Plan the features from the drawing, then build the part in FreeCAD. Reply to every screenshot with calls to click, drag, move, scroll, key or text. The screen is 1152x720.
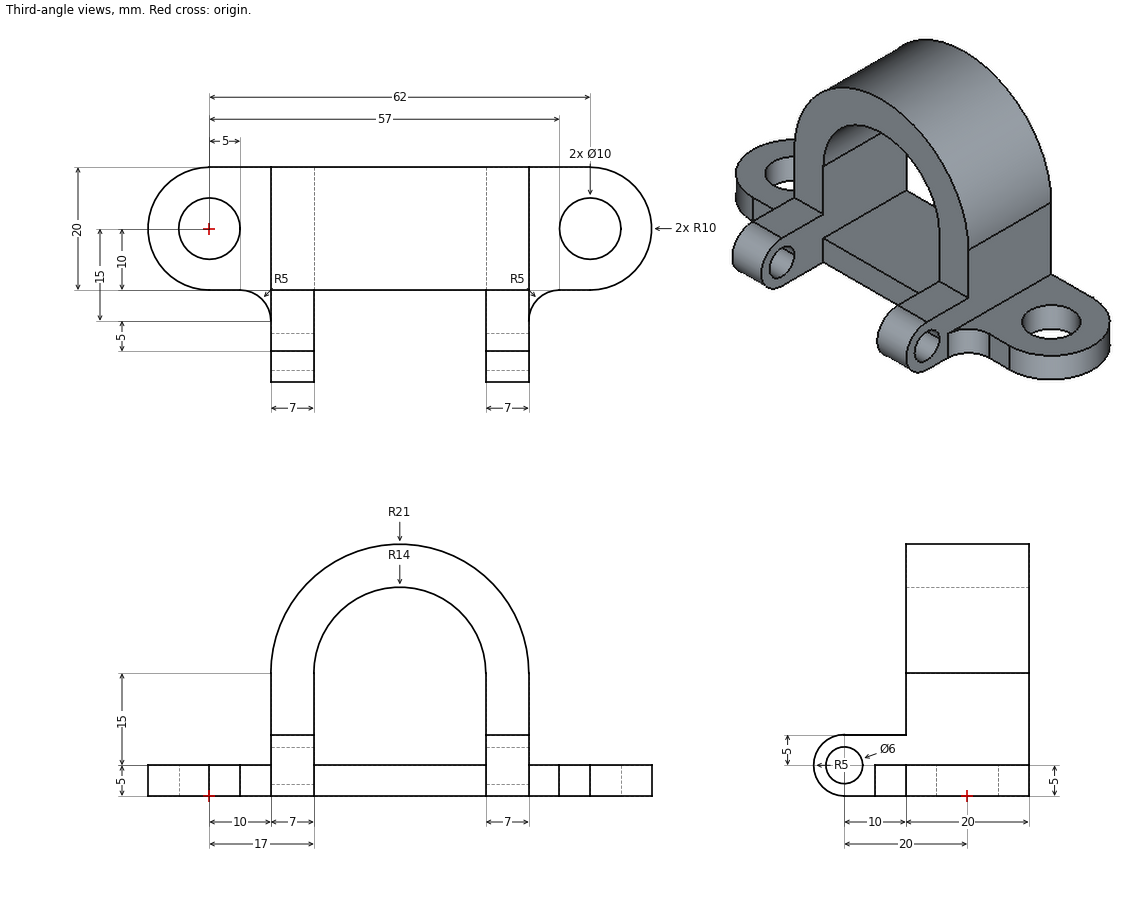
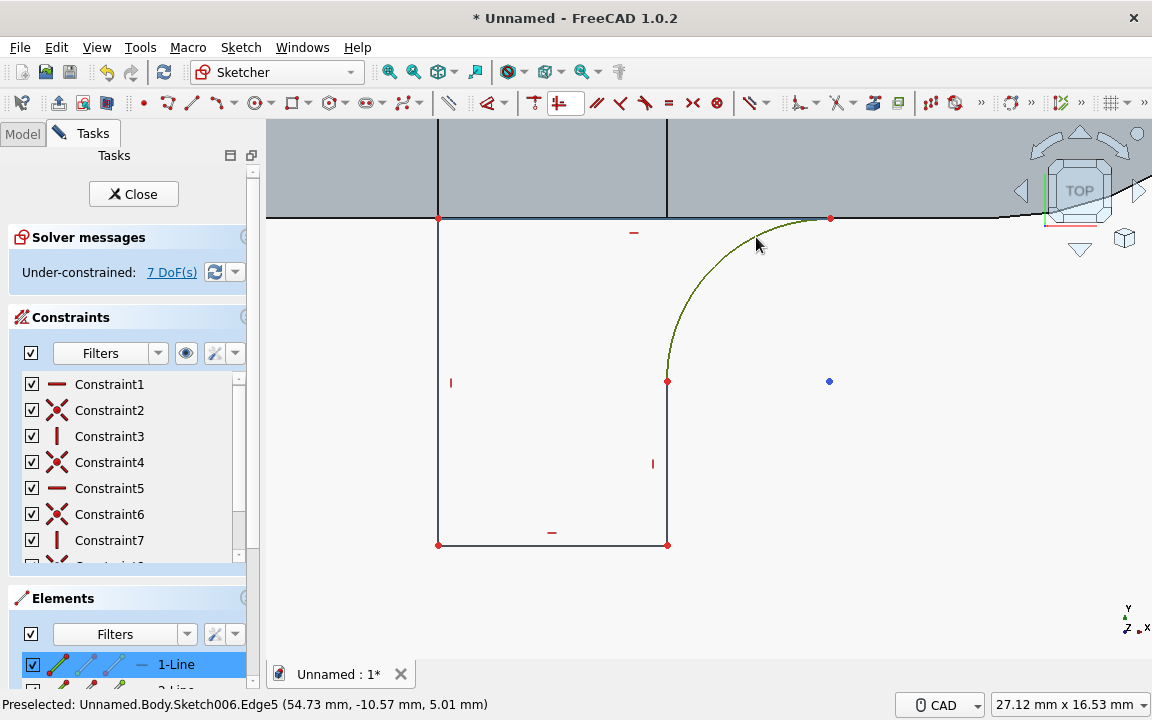
click(646, 104)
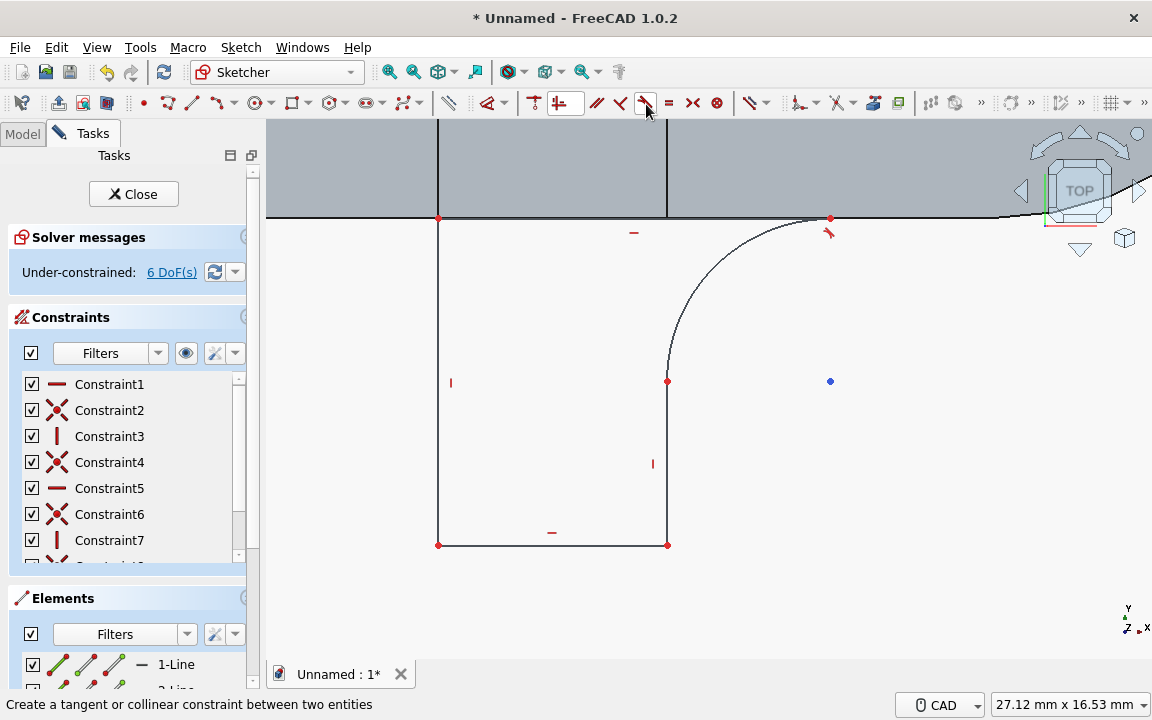
click(667, 497)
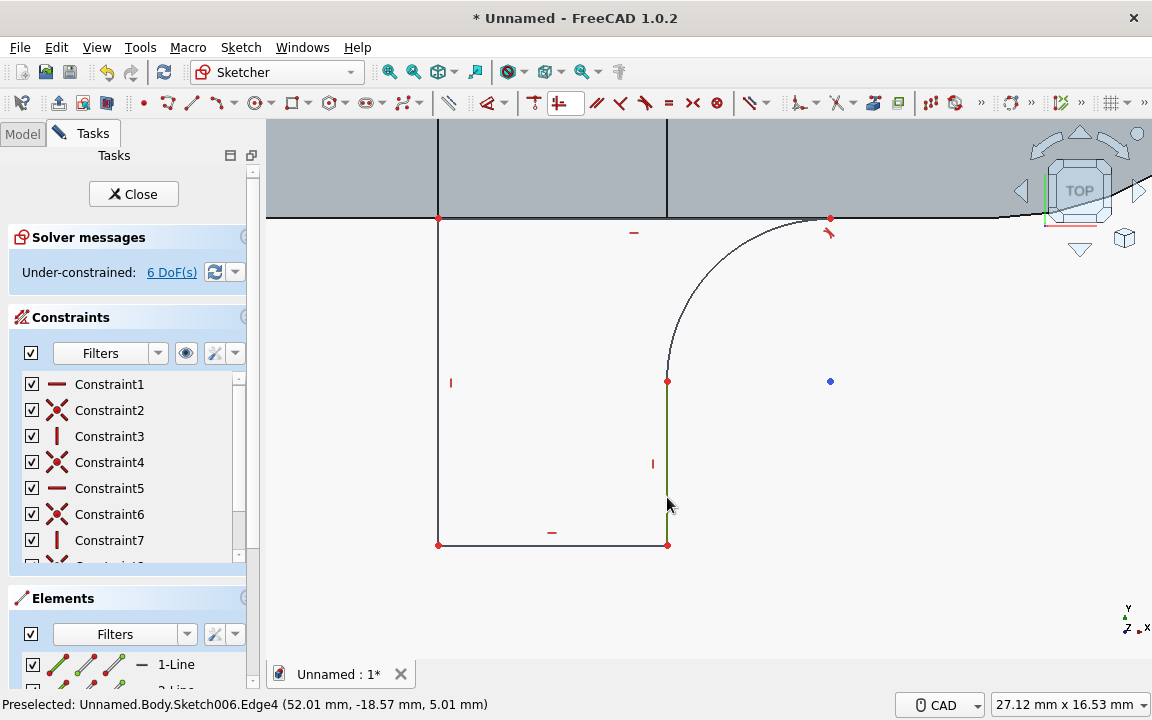
click(756, 237)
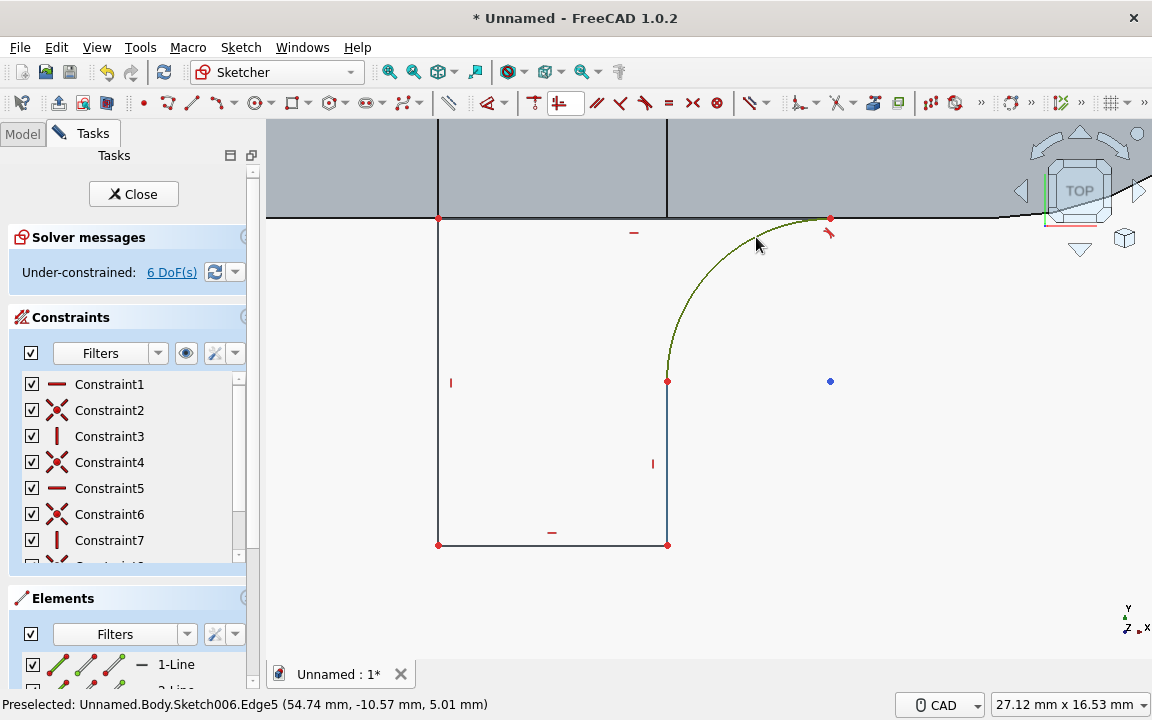
click(646, 104)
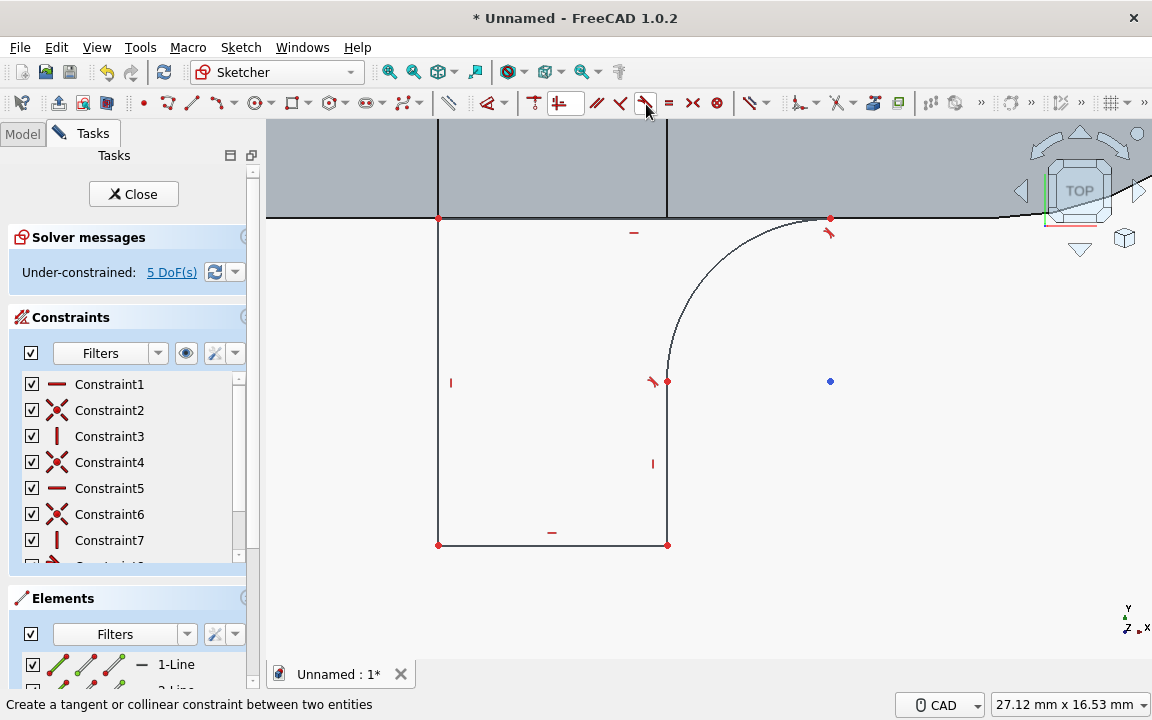
click(488, 104)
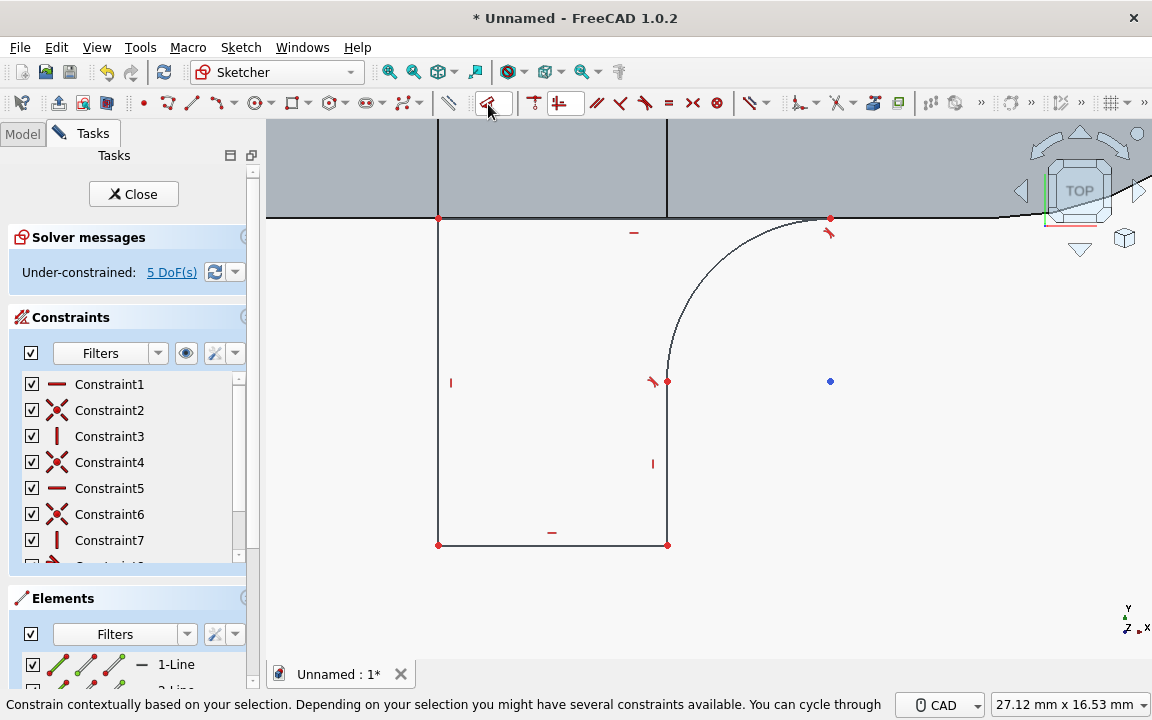
click(756, 237)
click(835, 187)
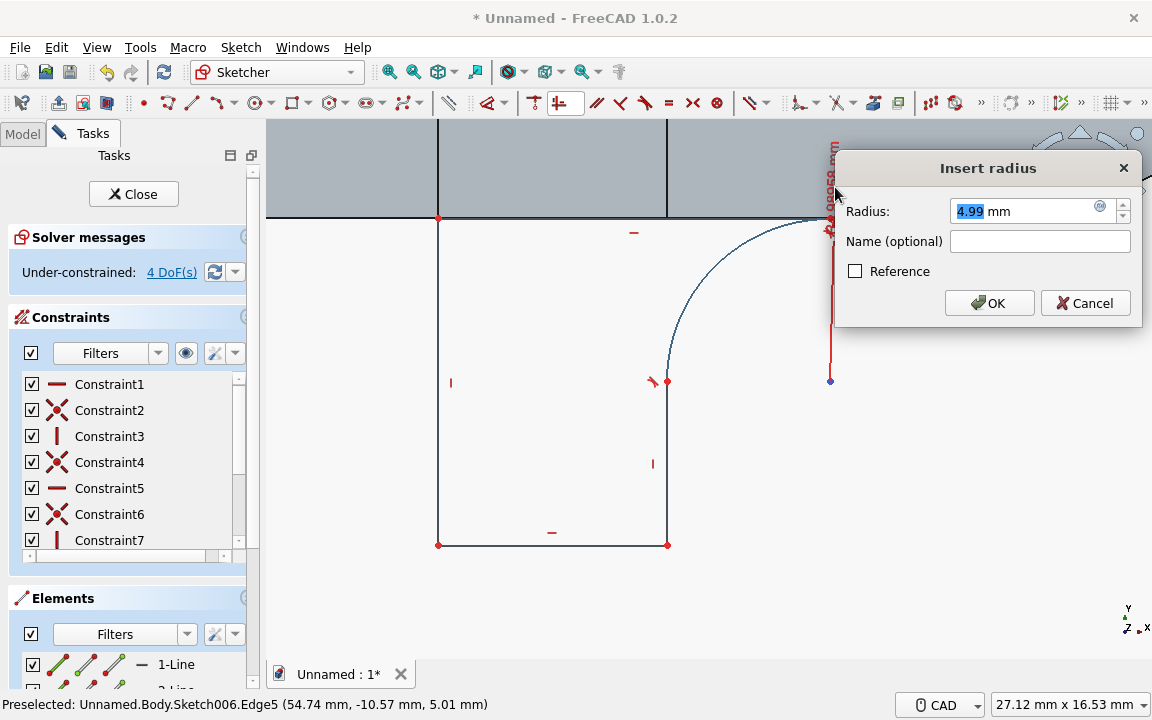
text(5)
key(Return)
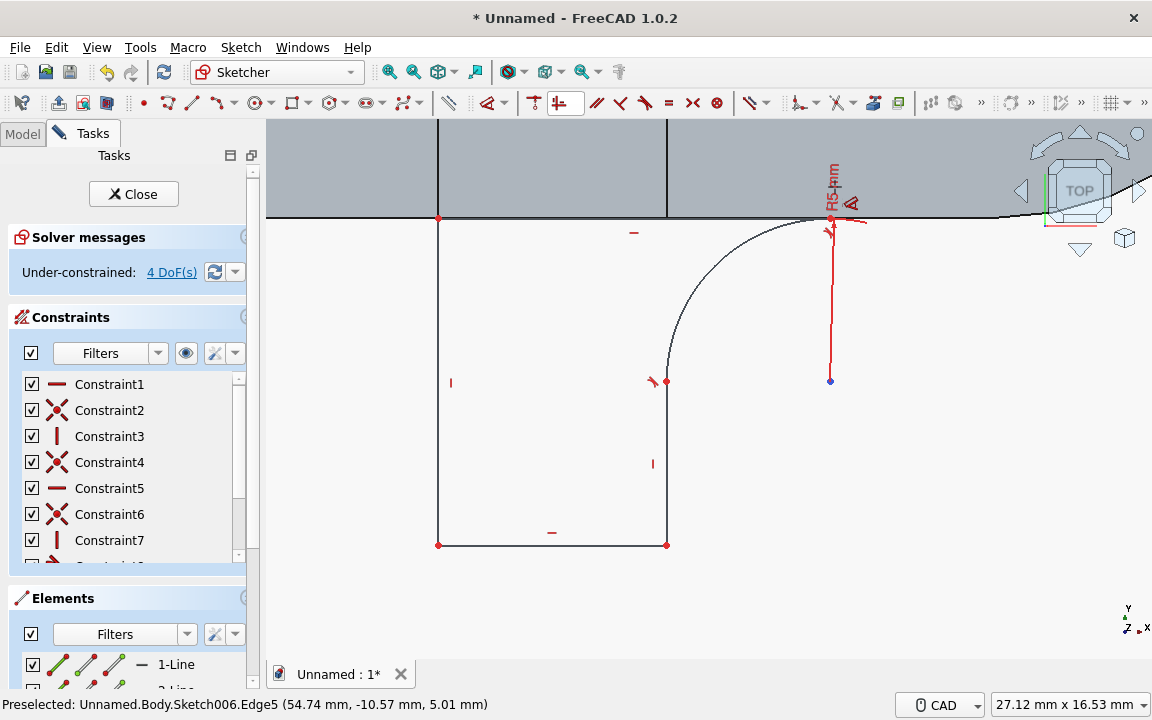
click(507, 546)
click(552, 580)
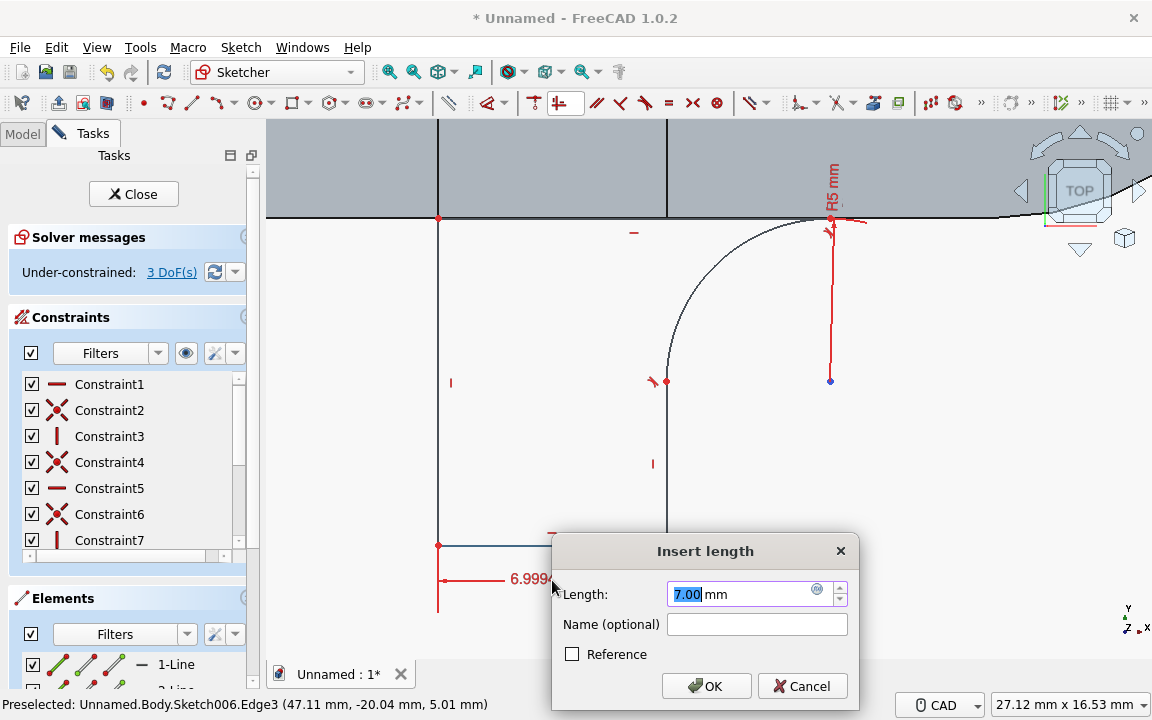
text(7)
key(Return)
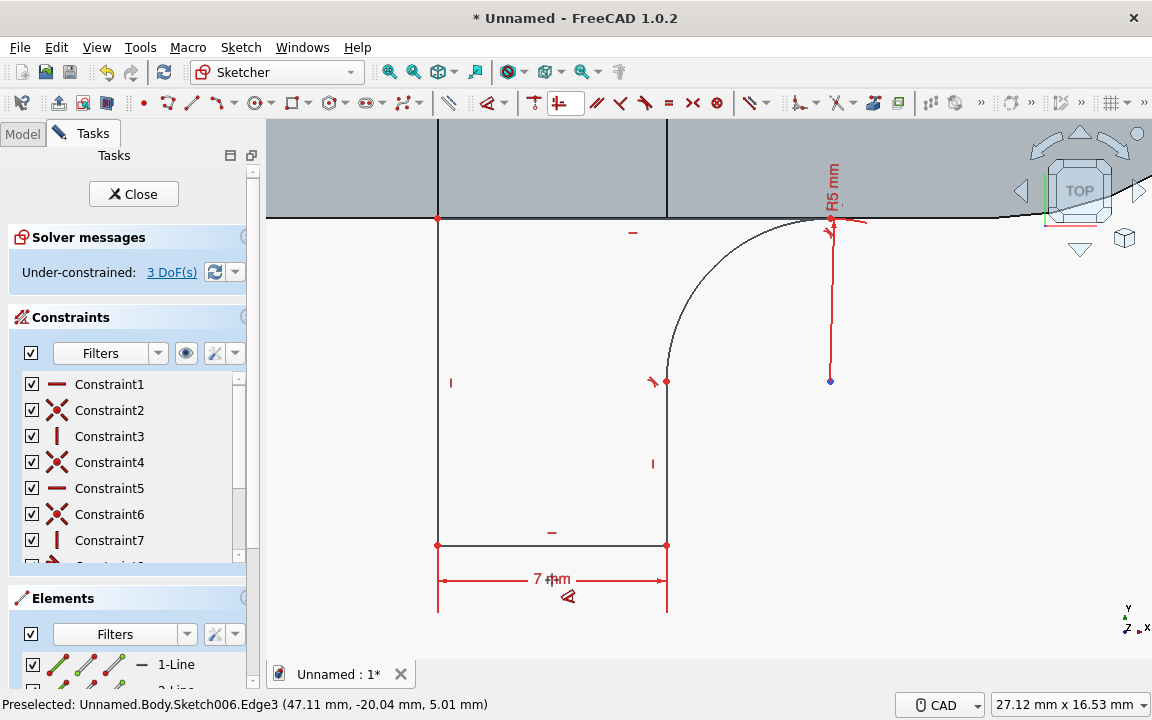
click(667, 497)
click(701, 464)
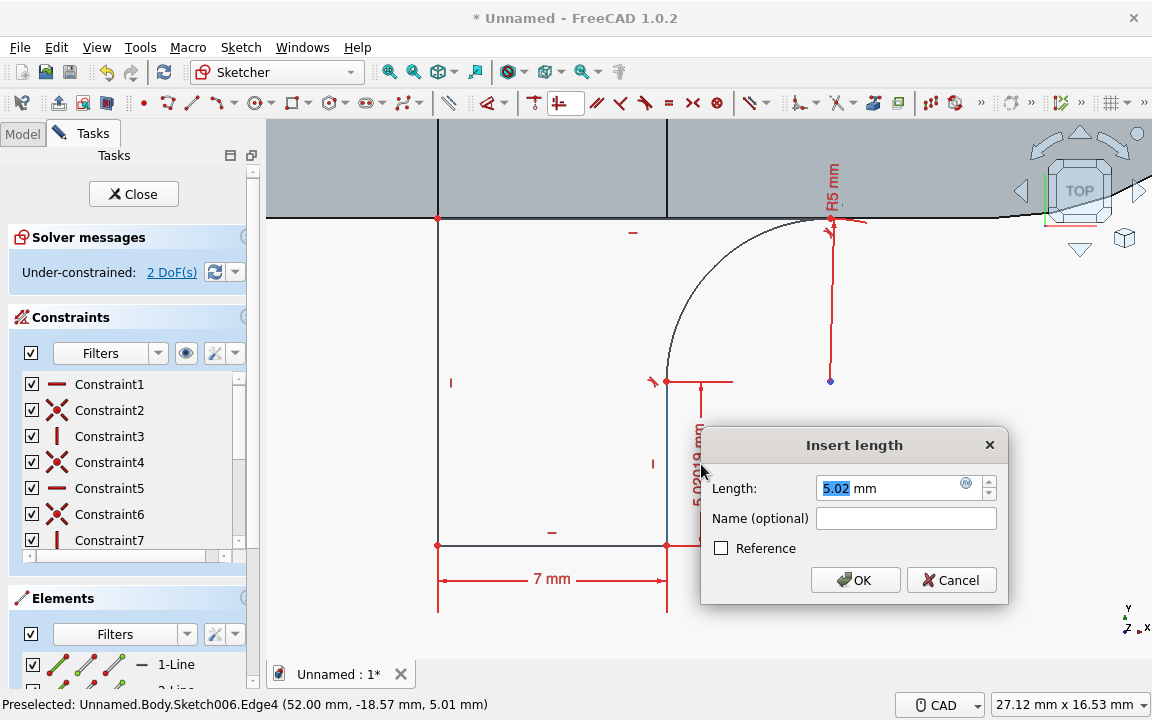
text(5)
key(Return)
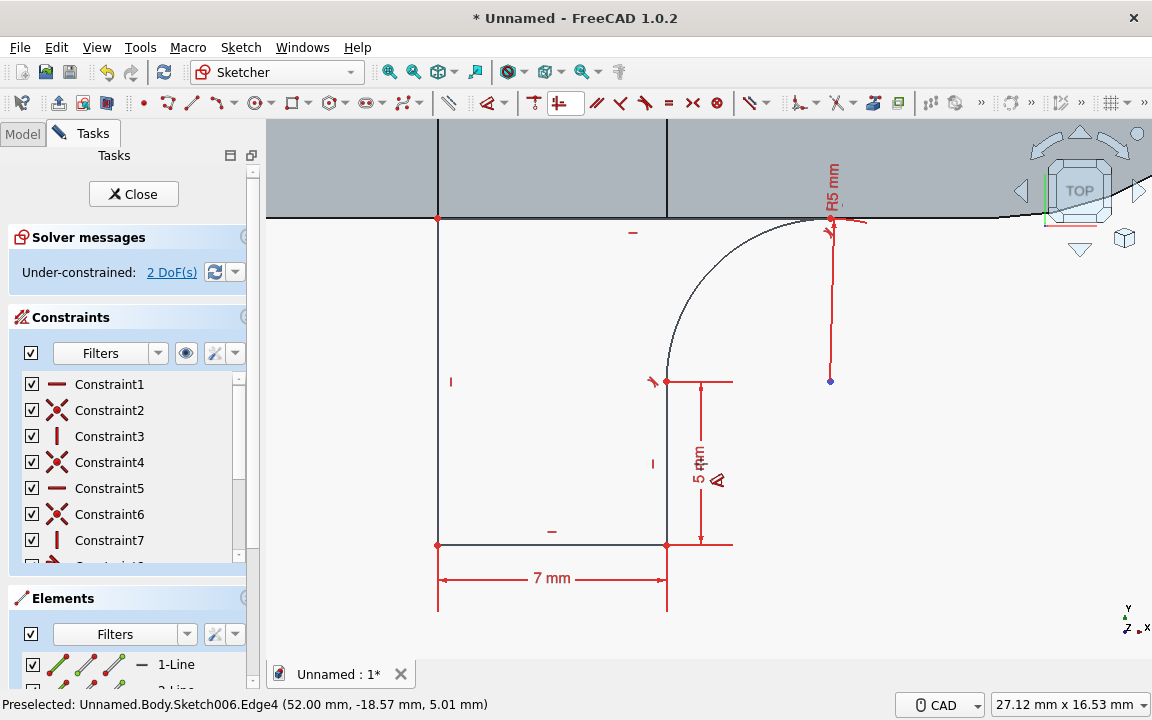
click(830, 219)
click(562, 253)